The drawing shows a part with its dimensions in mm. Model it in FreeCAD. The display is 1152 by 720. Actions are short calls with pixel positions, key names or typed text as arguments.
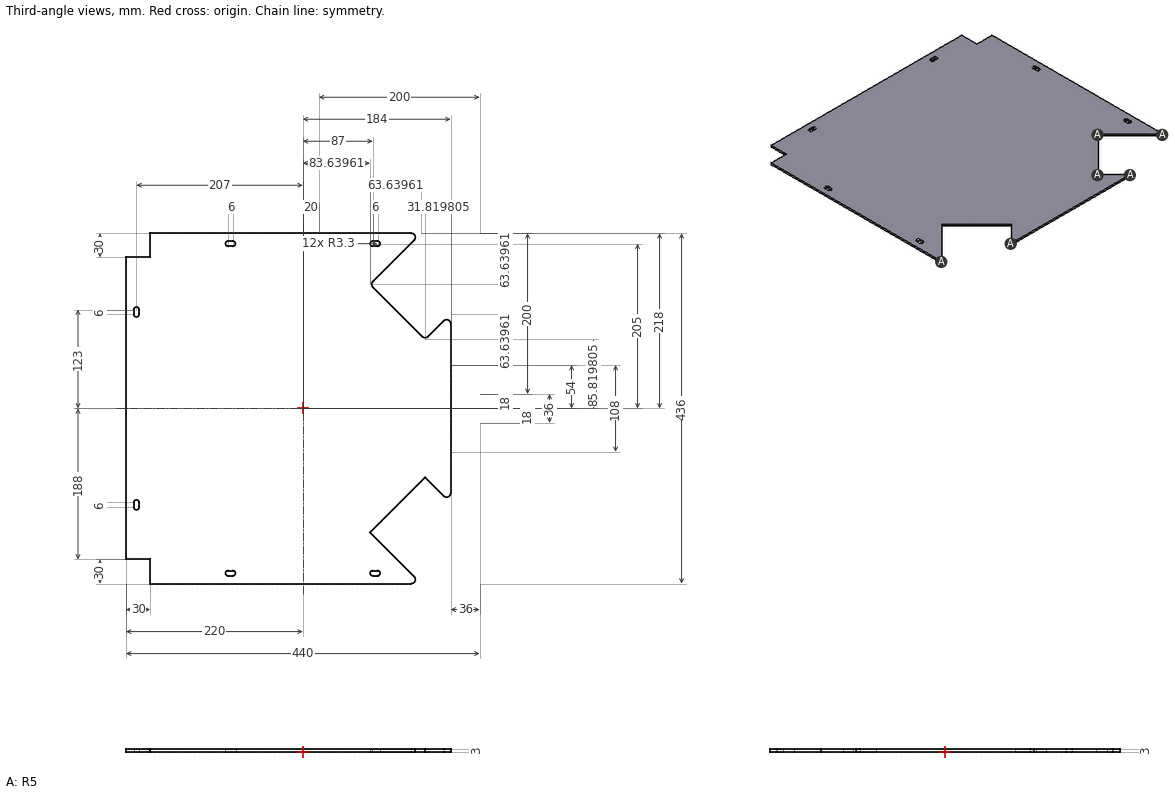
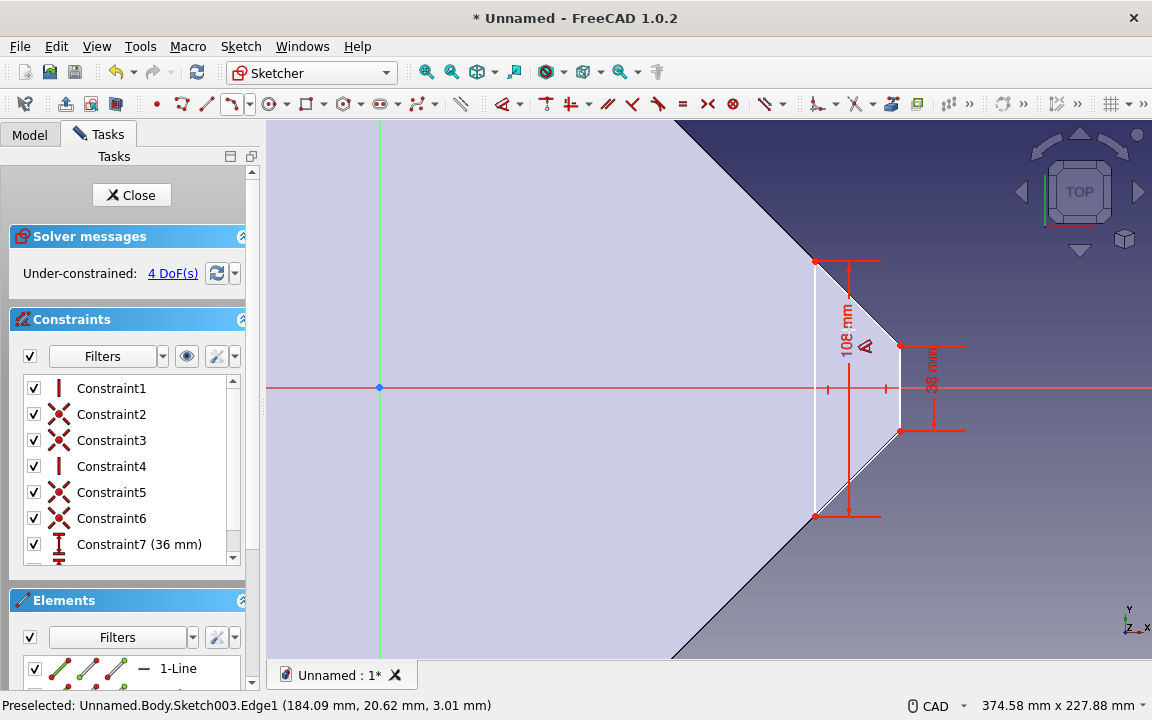
click(815, 261)
click(346, 325)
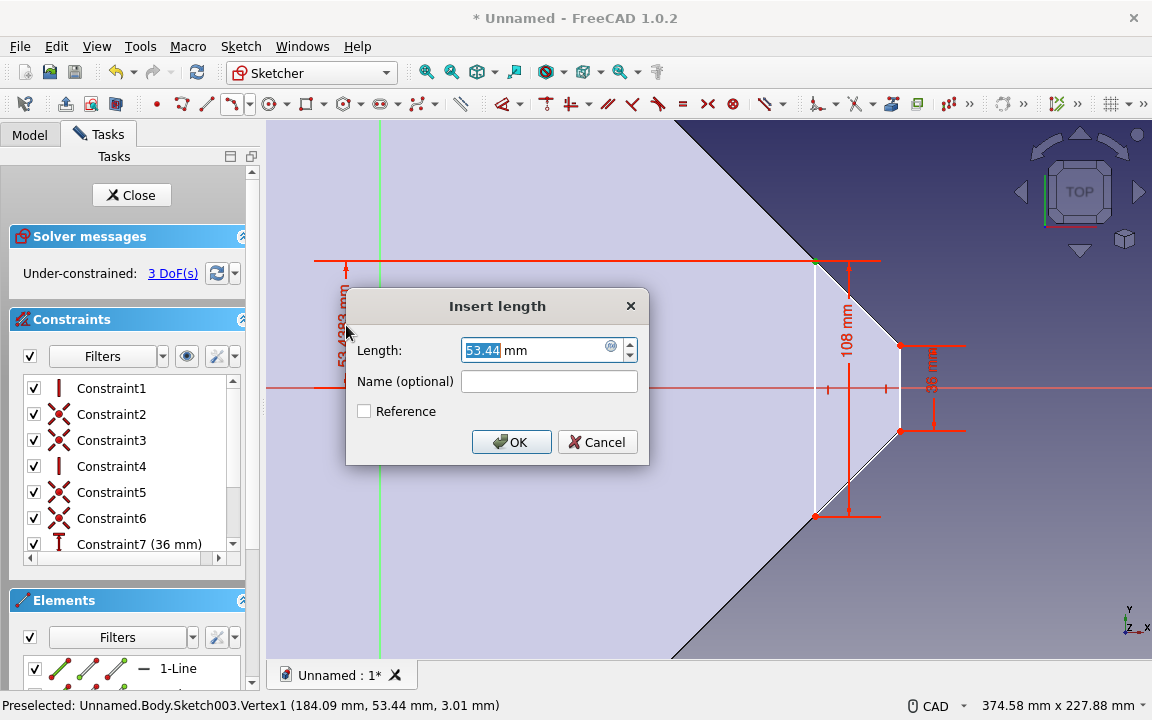
text(54)
key(Return)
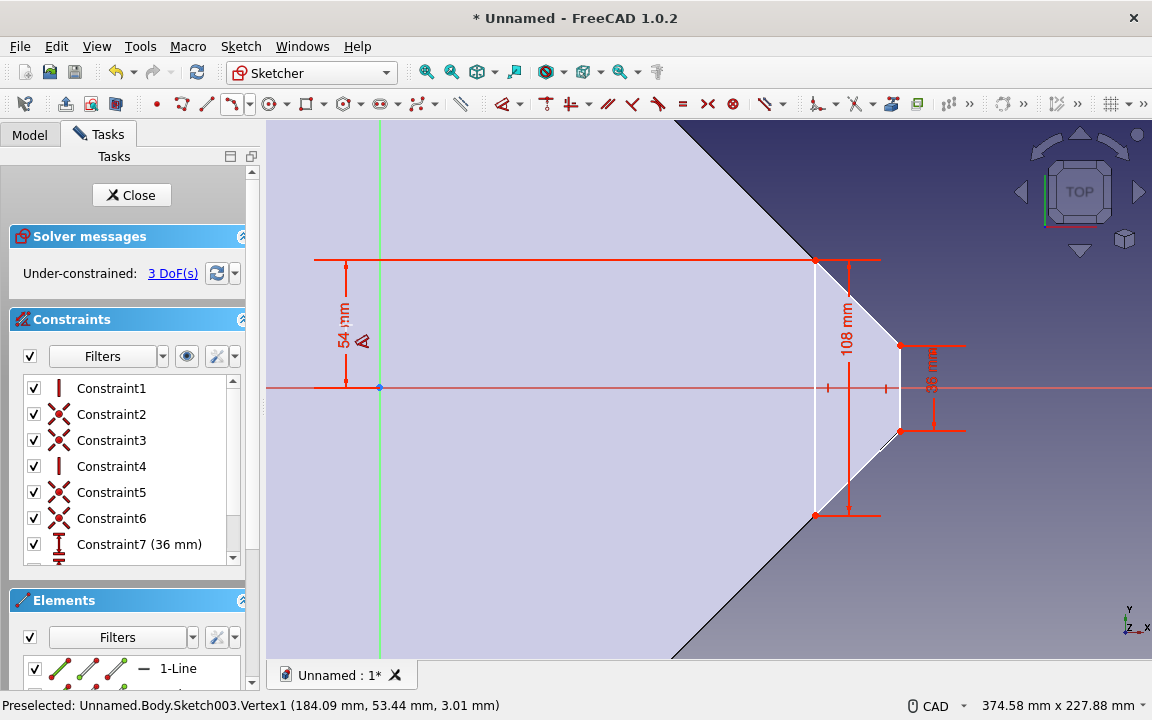
click(900, 431)
click(934, 409)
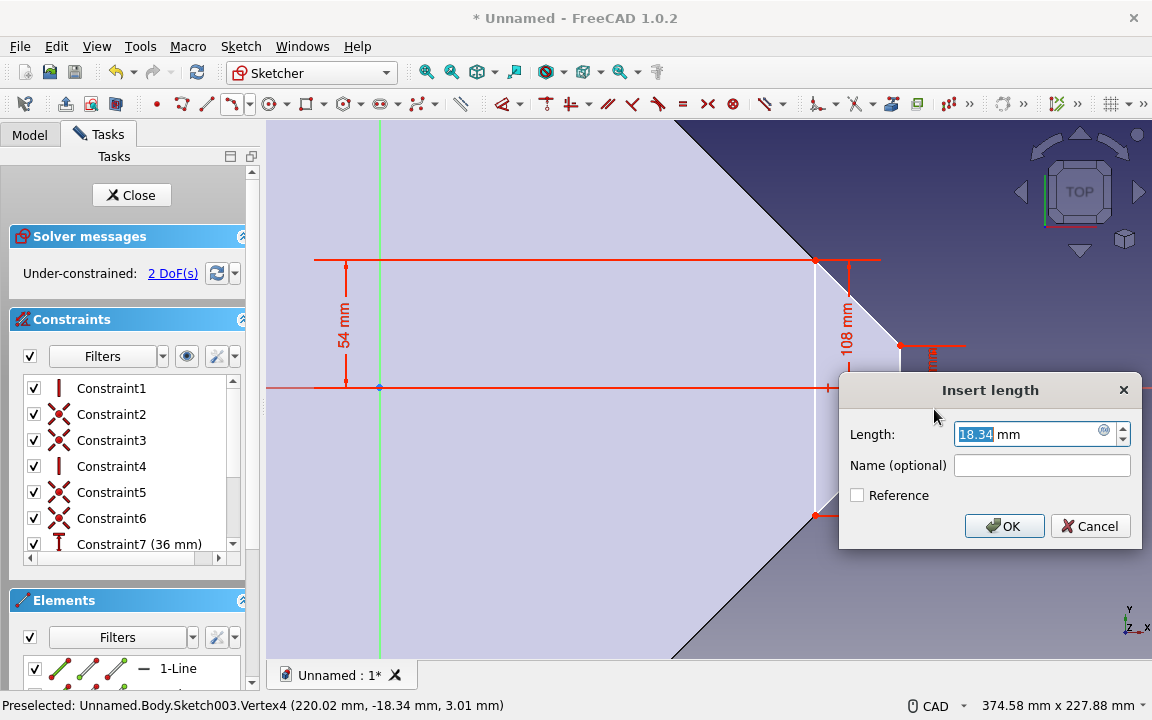
text(18)
key(Return)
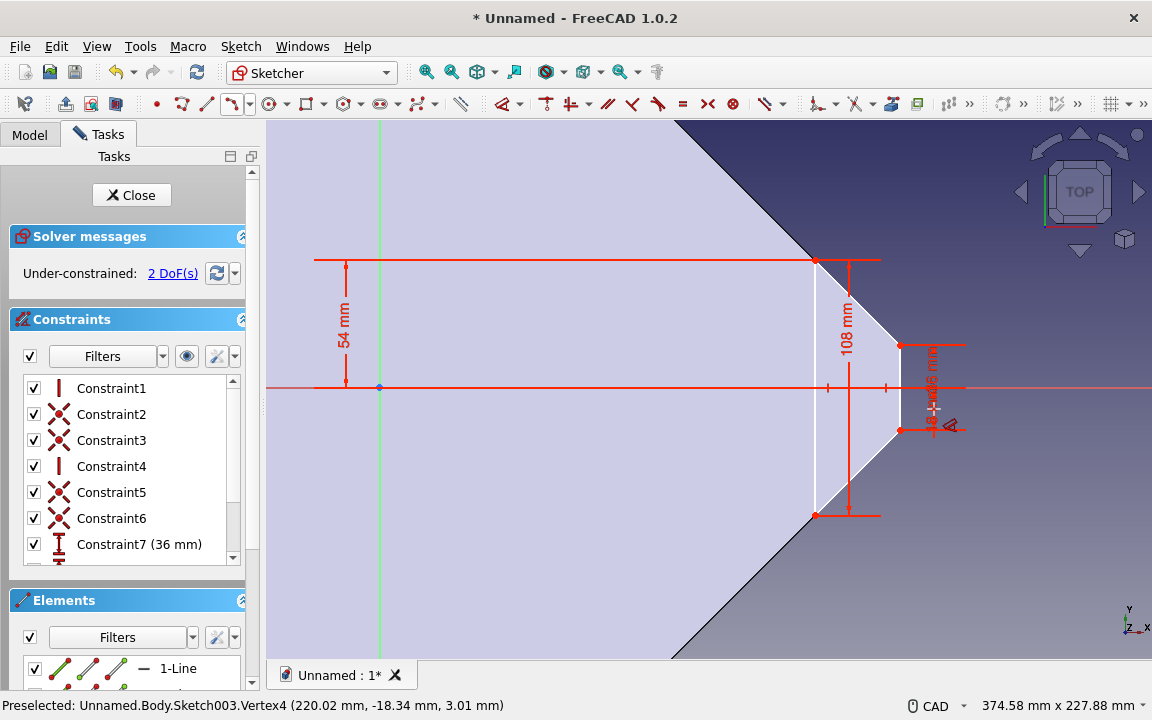
click(841, 490)
click(858, 550)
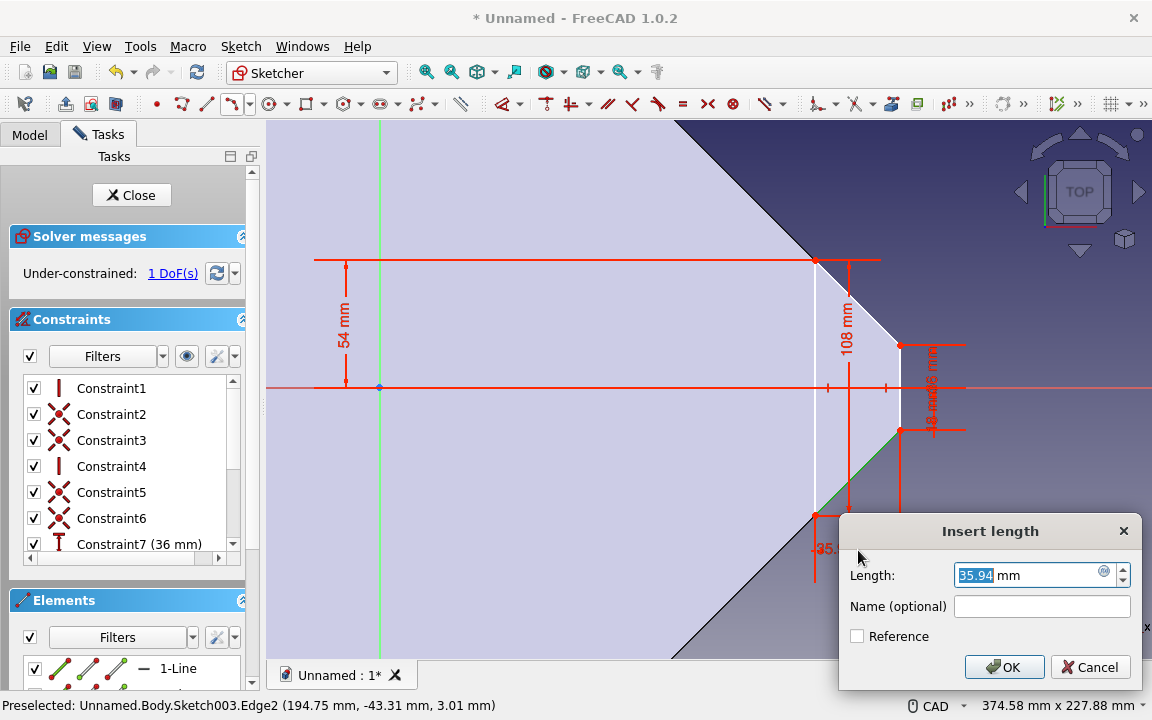
text(36)
key(Return)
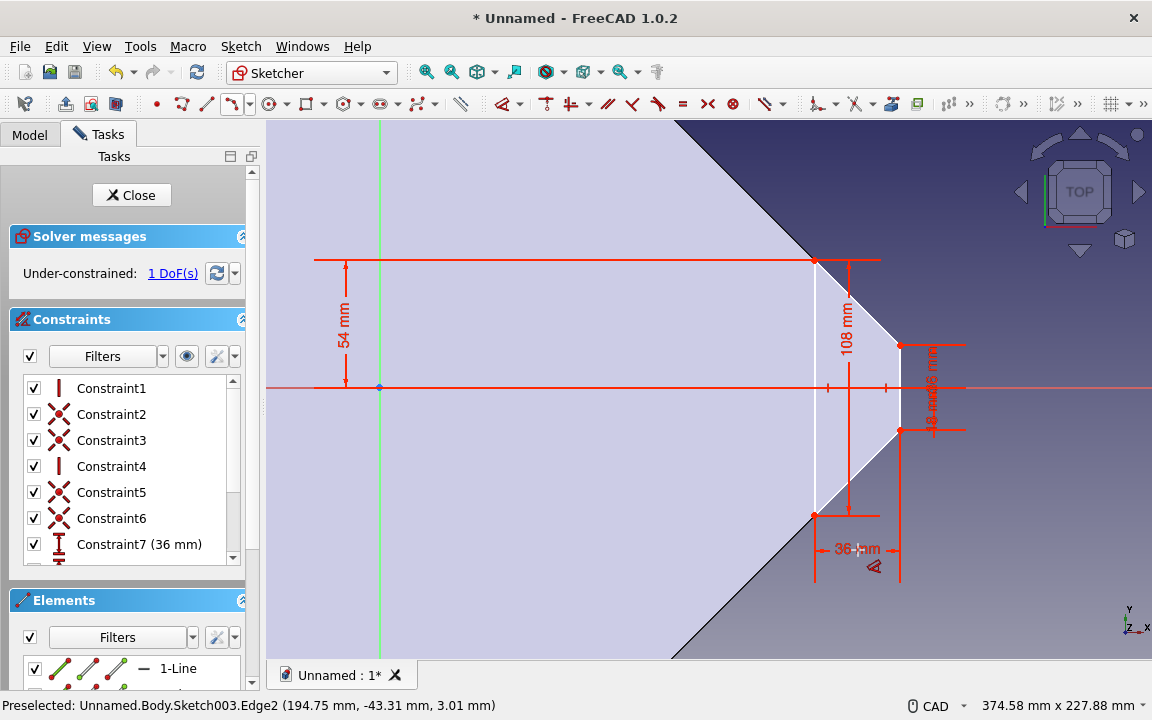
click(815, 260)
click(597, 226)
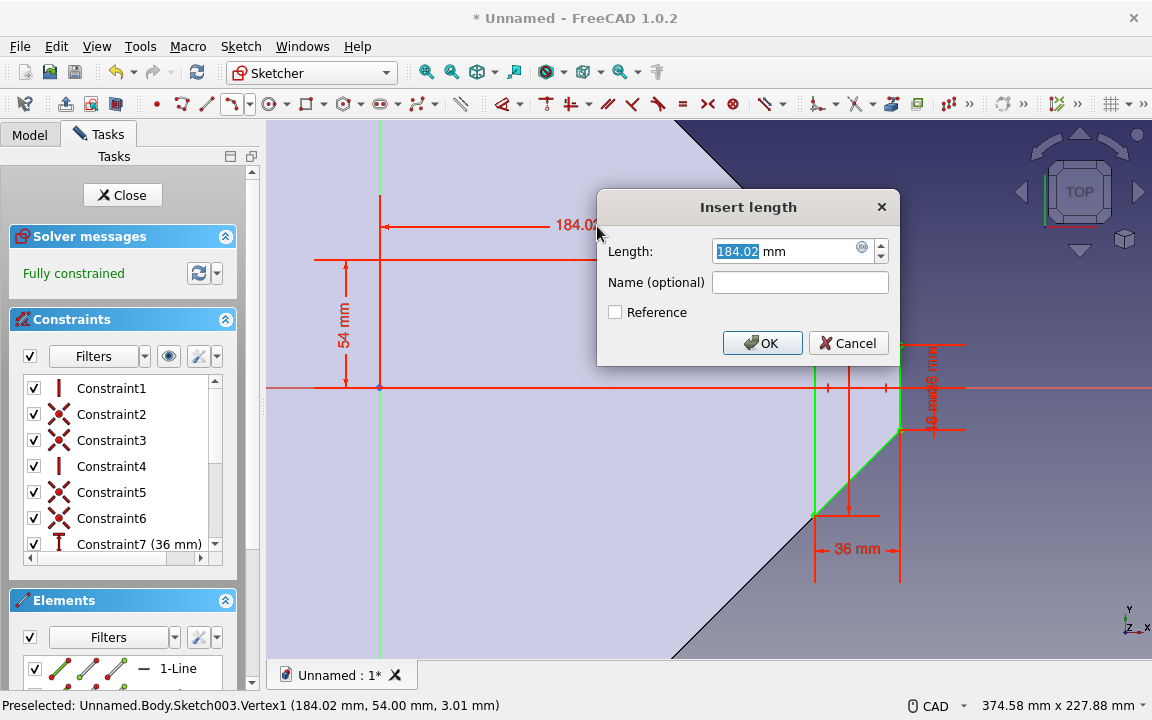
text(184)
key(Return)
key(Escape)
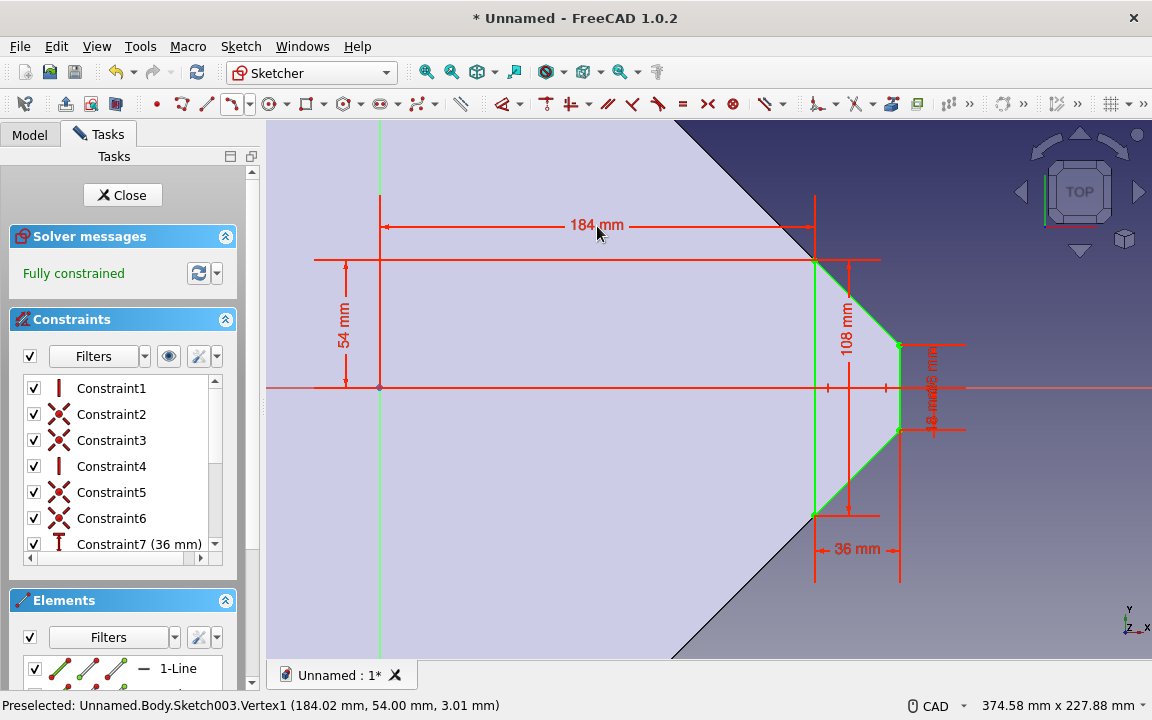
click(123, 195)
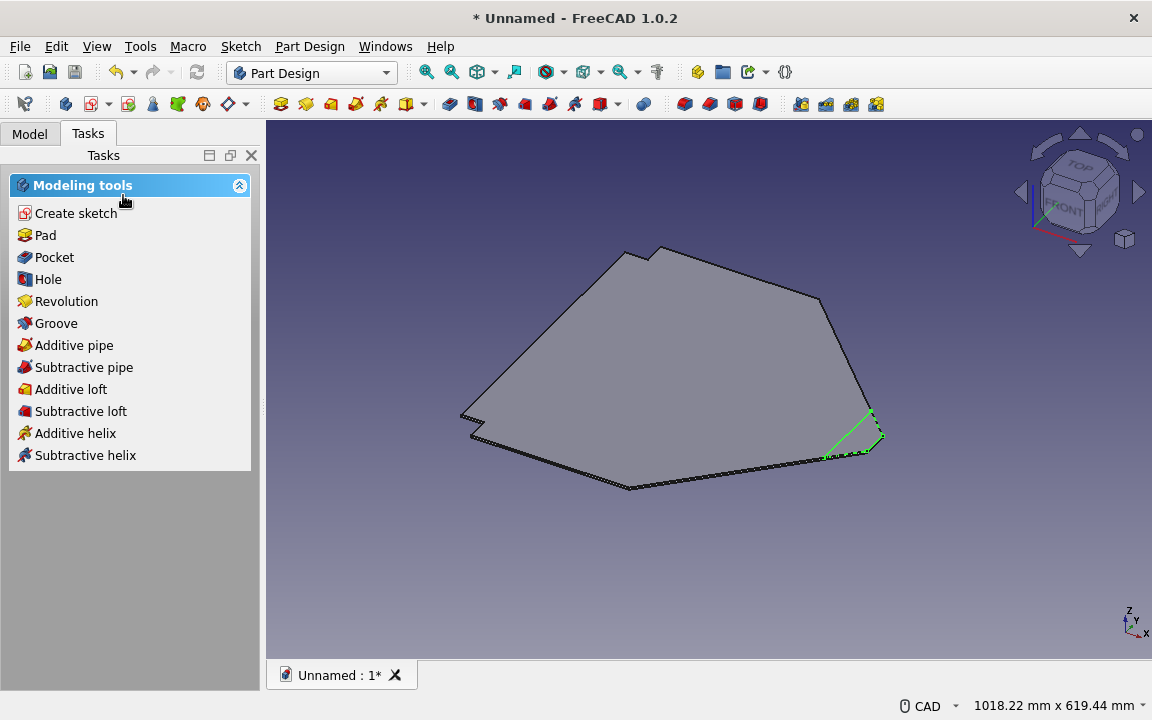
click(450, 104)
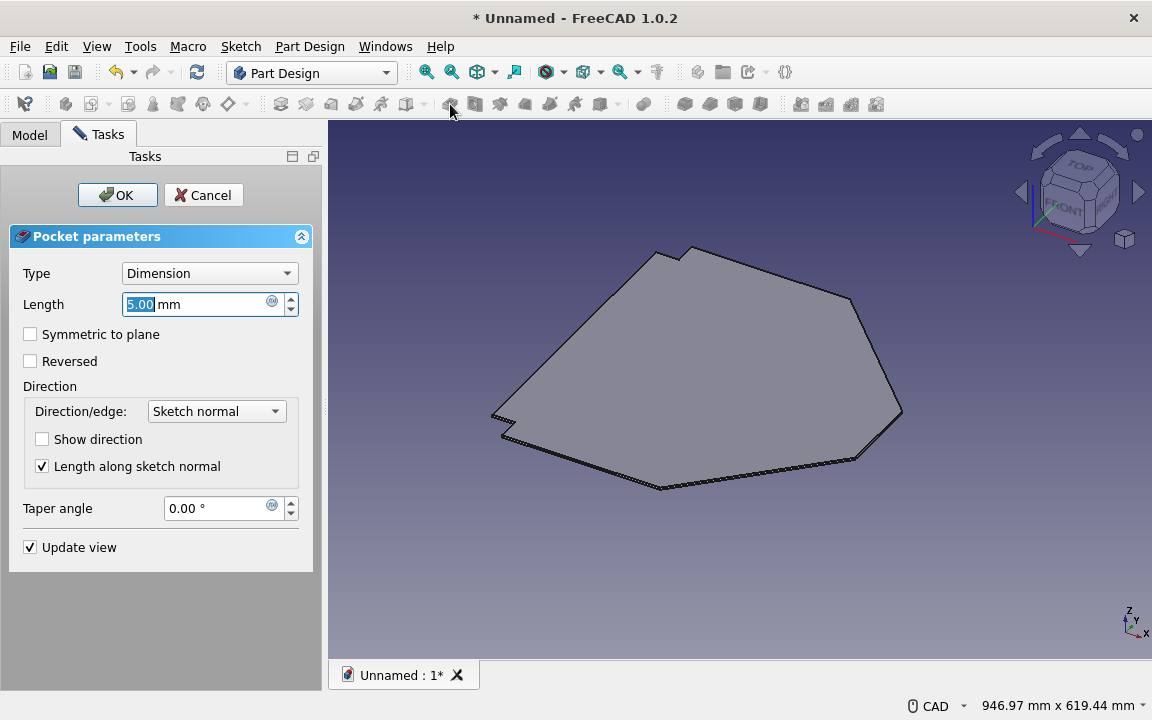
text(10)
key(Tab)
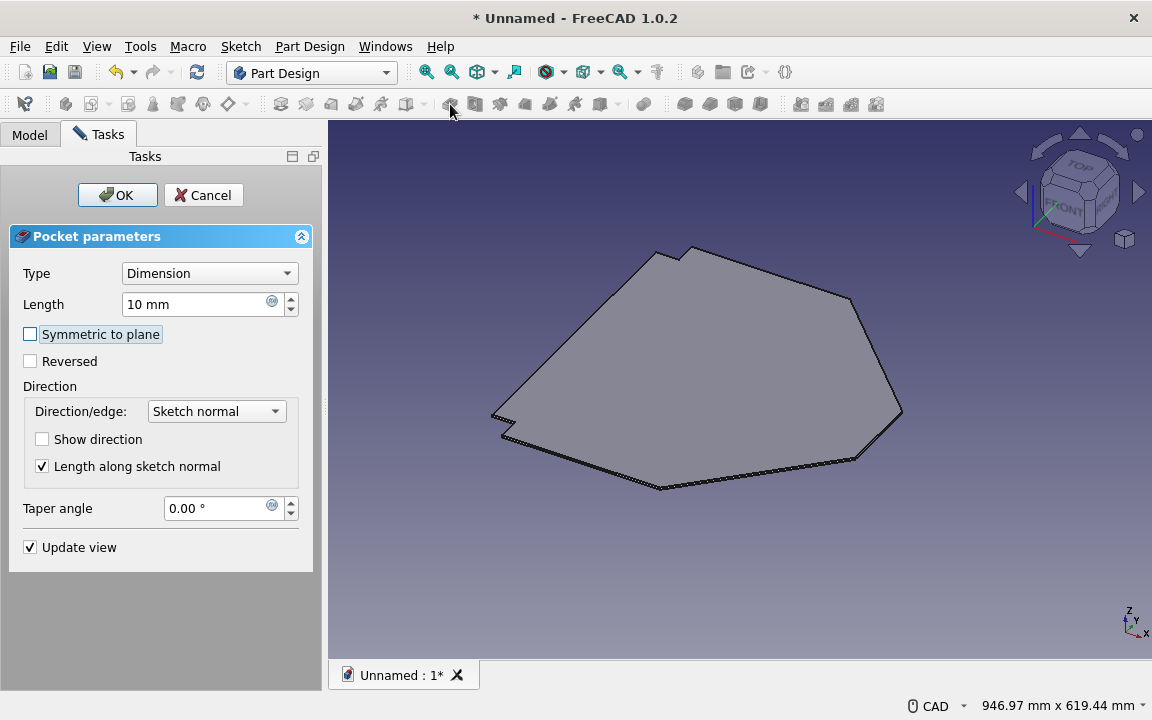
click(118, 195)